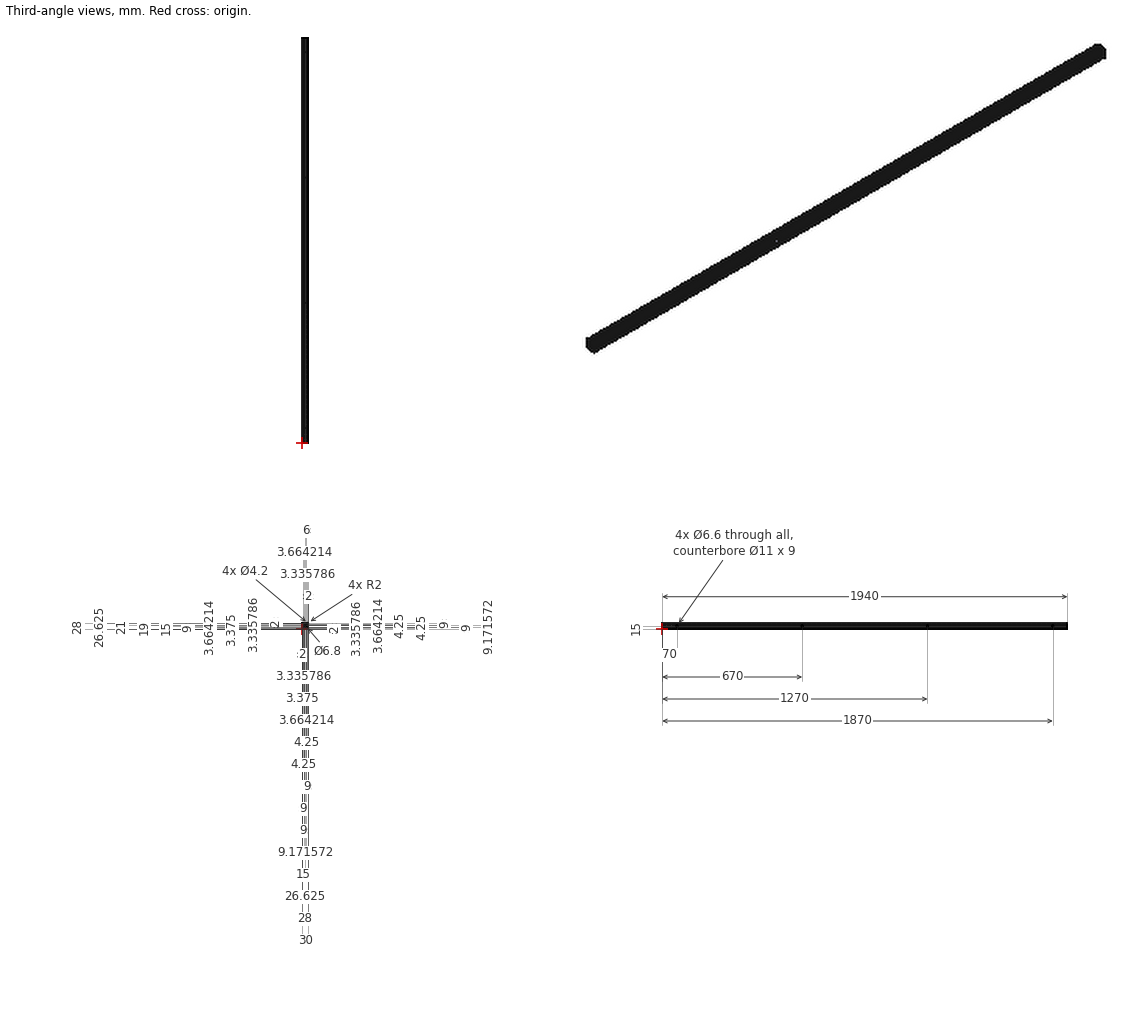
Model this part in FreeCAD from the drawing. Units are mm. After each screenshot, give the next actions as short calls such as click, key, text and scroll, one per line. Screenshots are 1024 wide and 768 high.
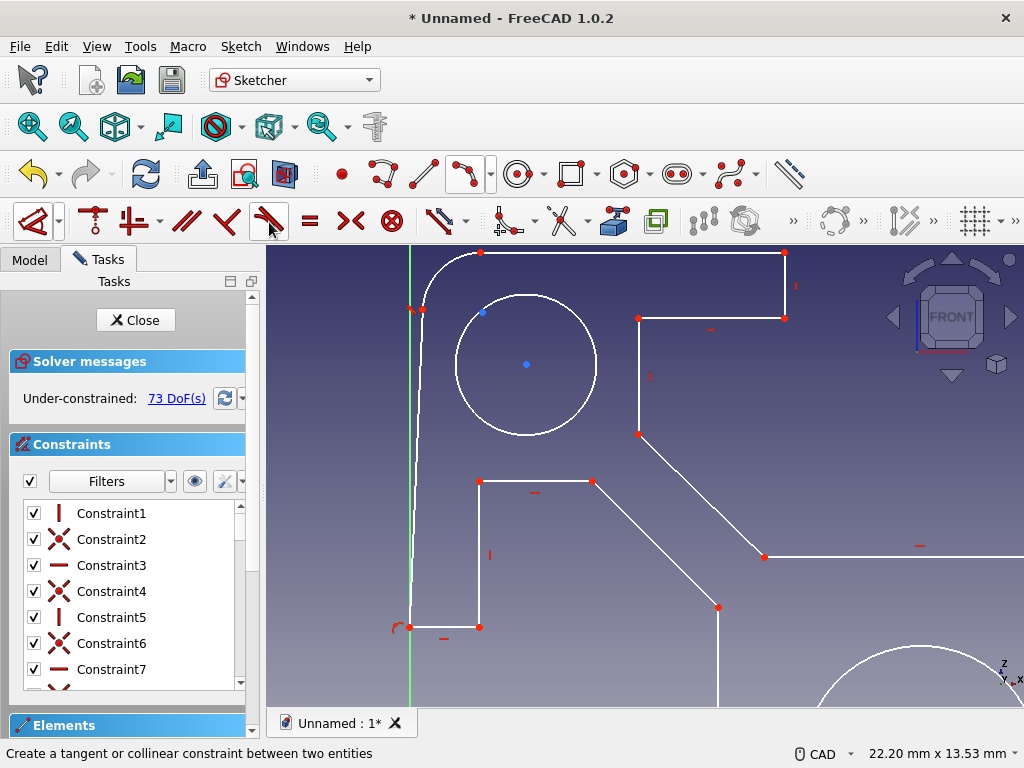
scroll(428, 354, down, 6)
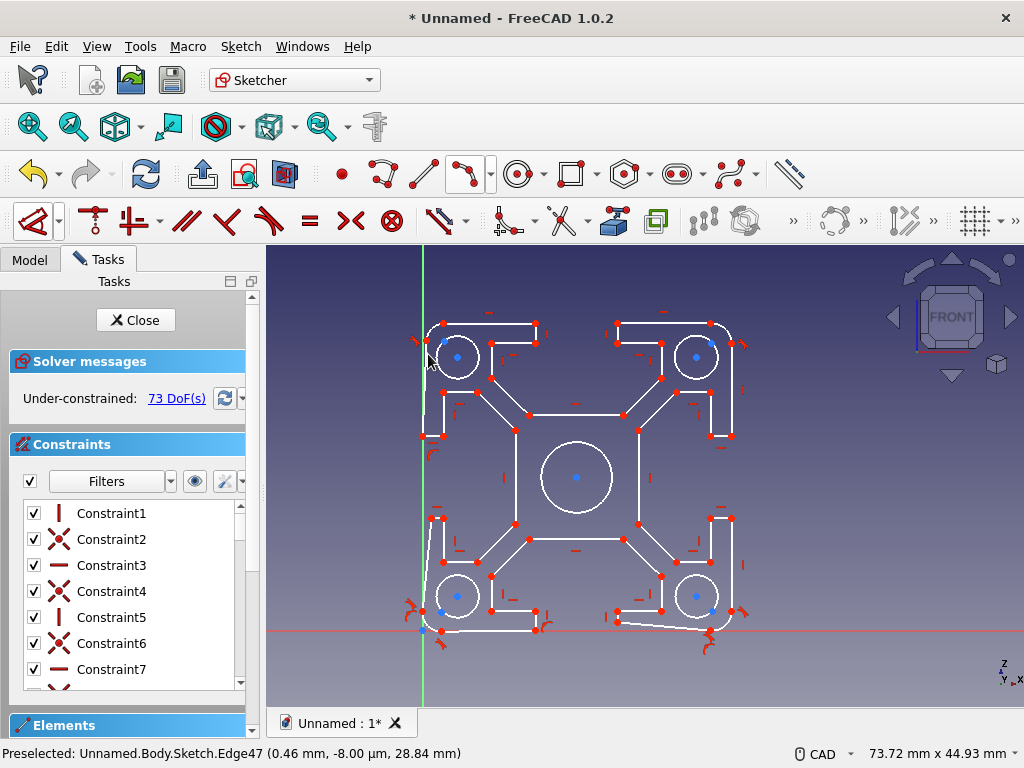
click(471, 324)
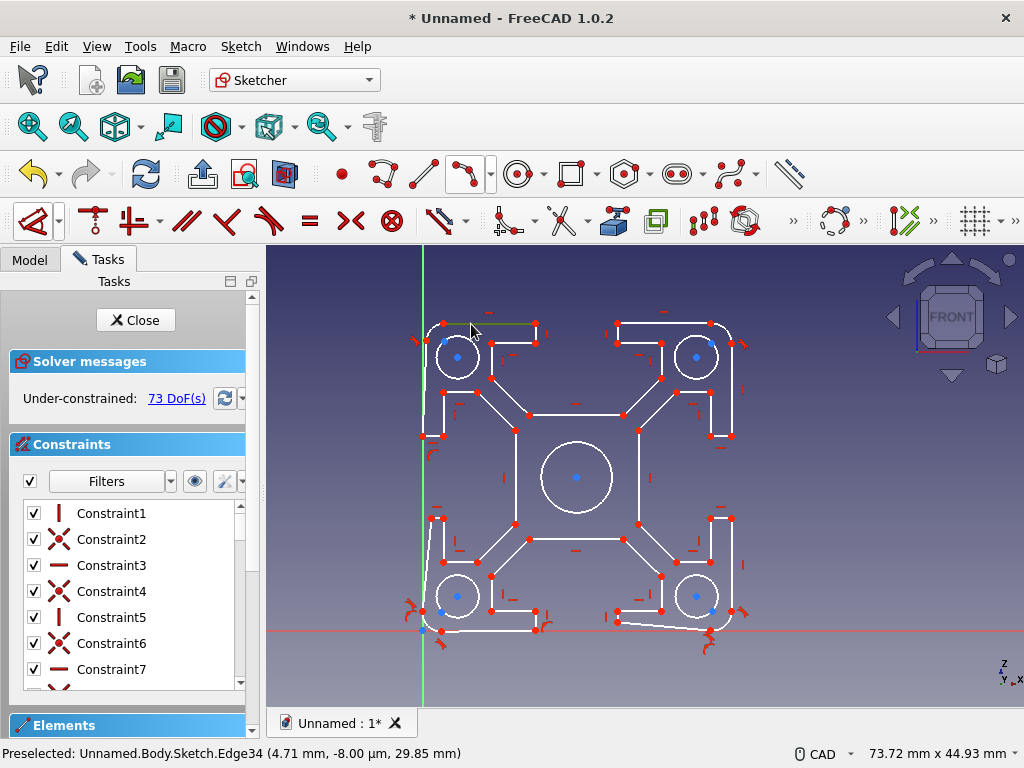
scroll(432, 329, up, 2)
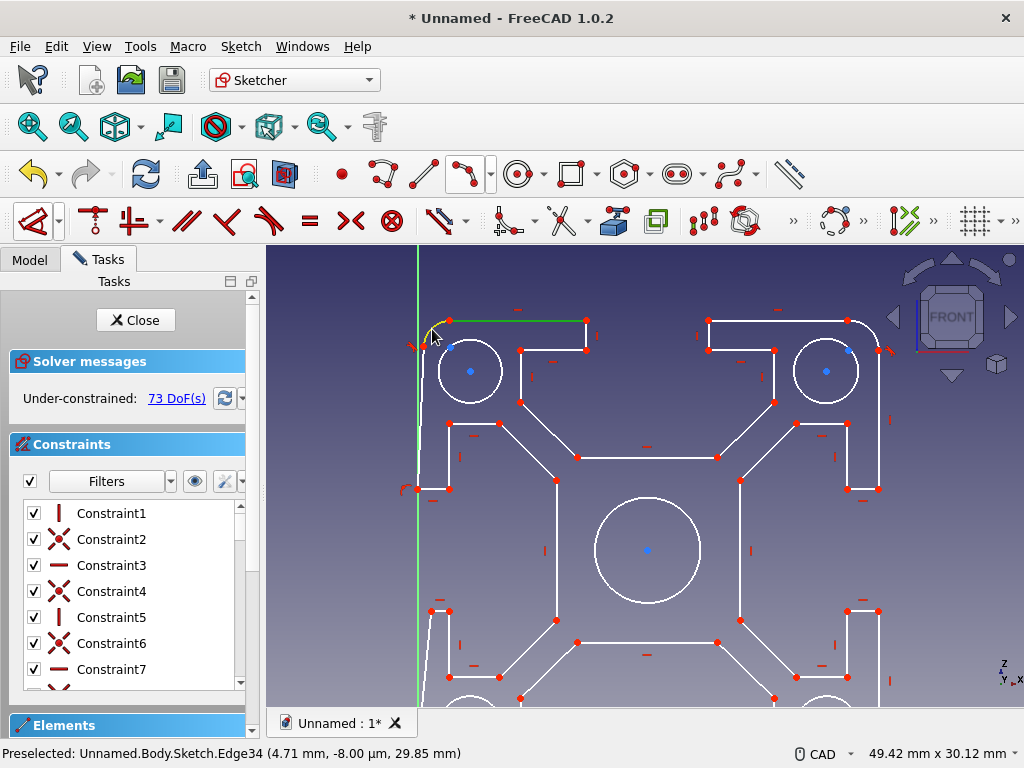
click(432, 329)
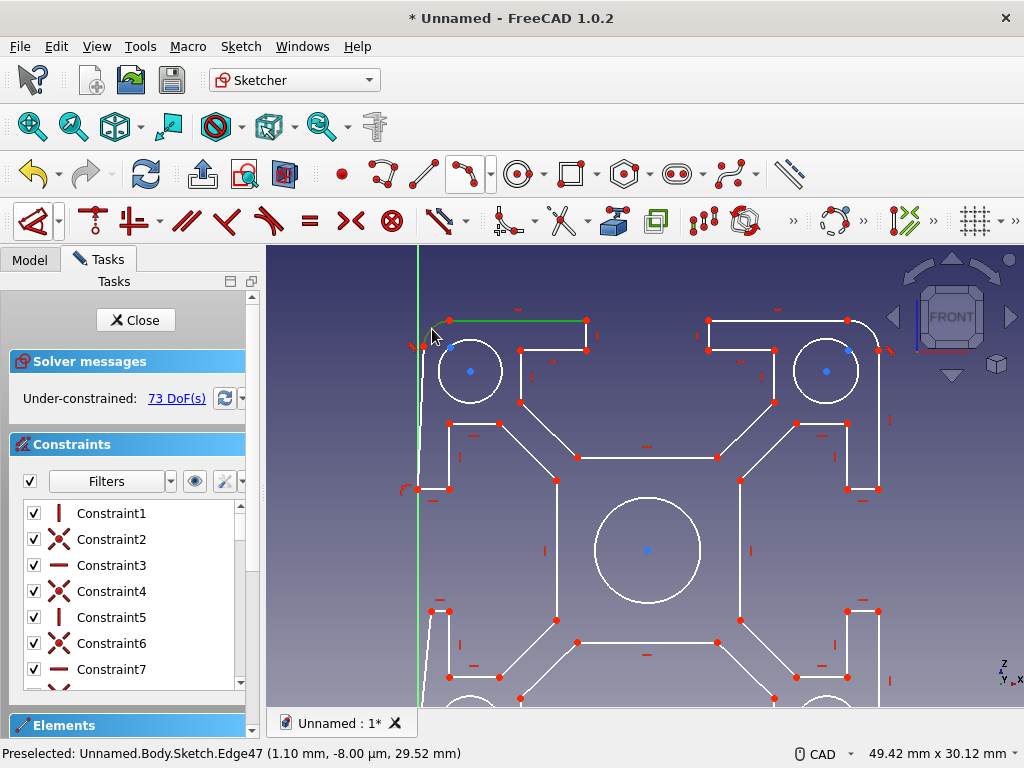
click(269, 222)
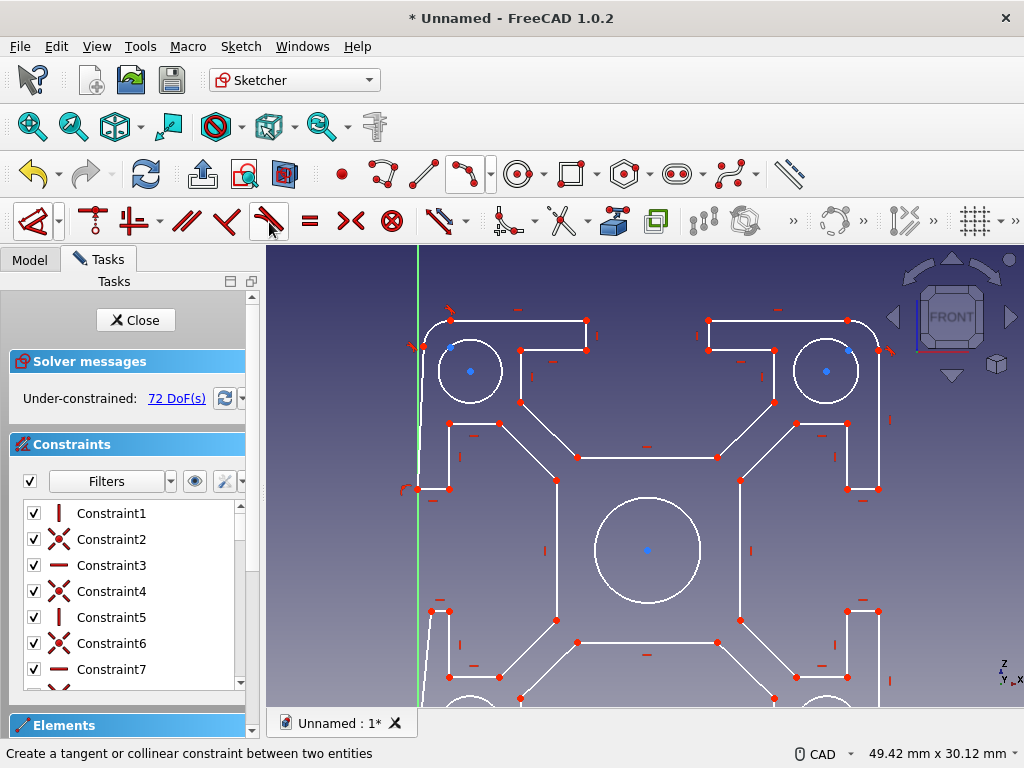
click(750, 321)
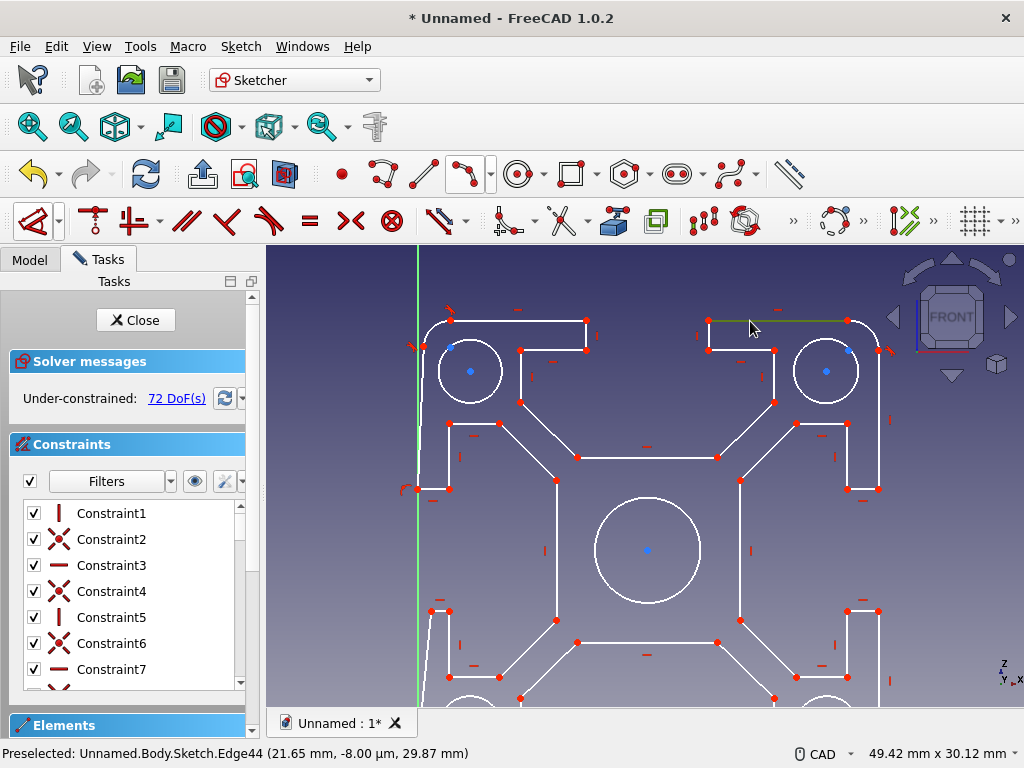
scroll(857, 322, up, 2)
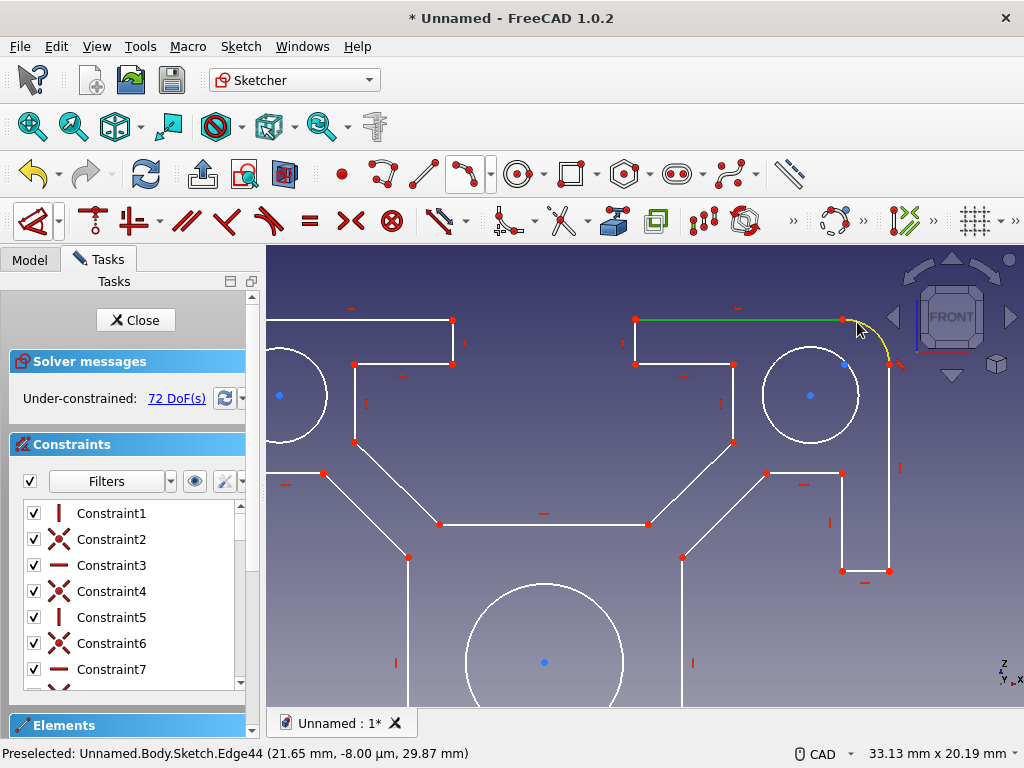
click(857, 321)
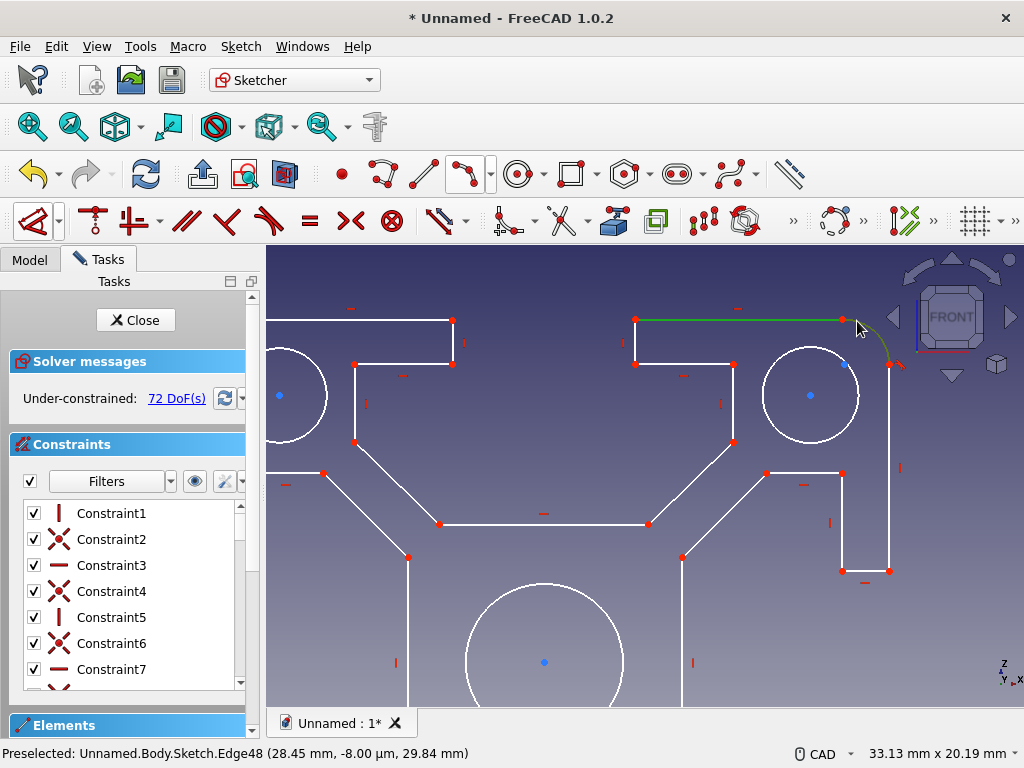
key(t)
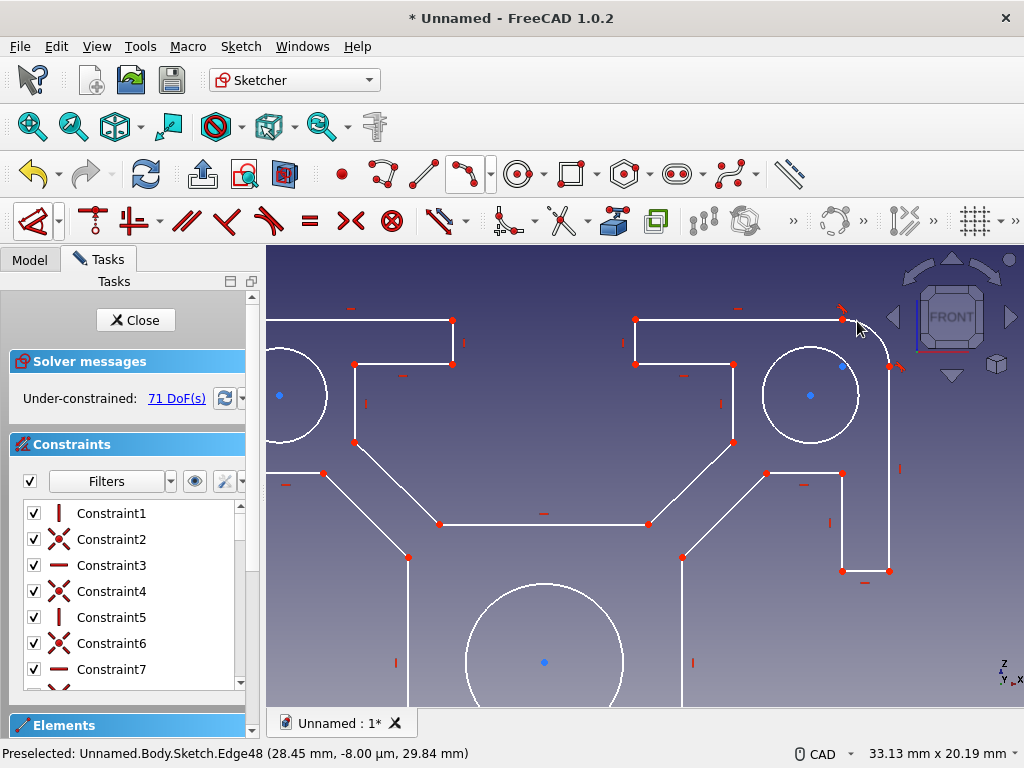
scroll(602, 326, down, 4)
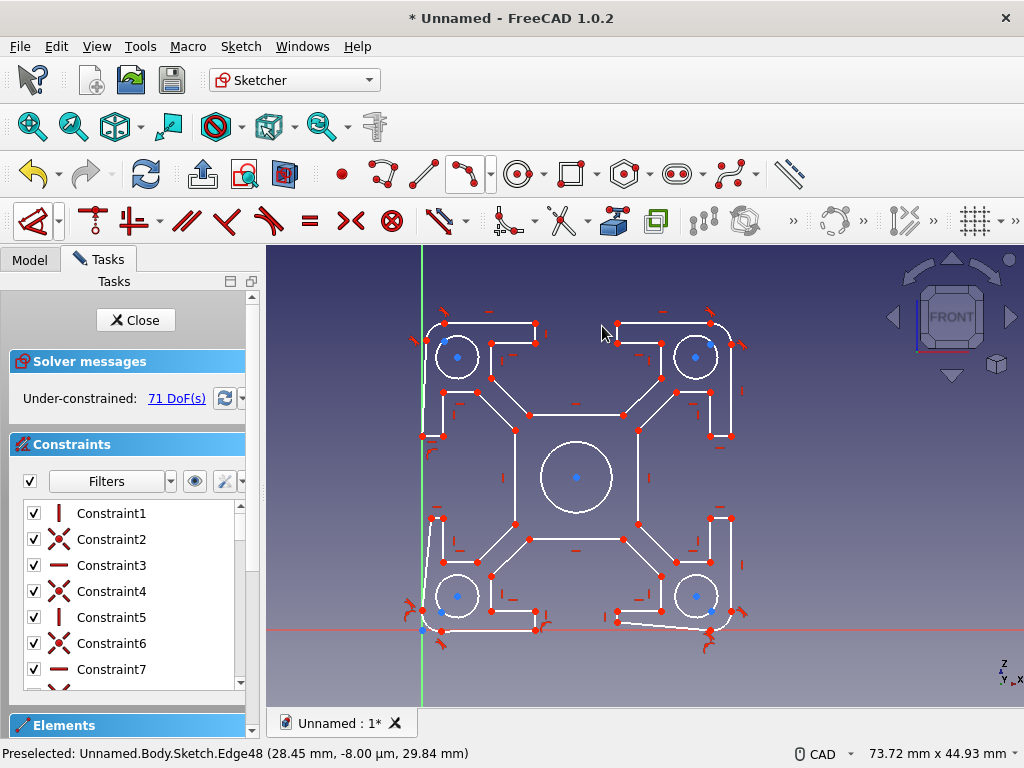
scroll(645, 625, up, 5)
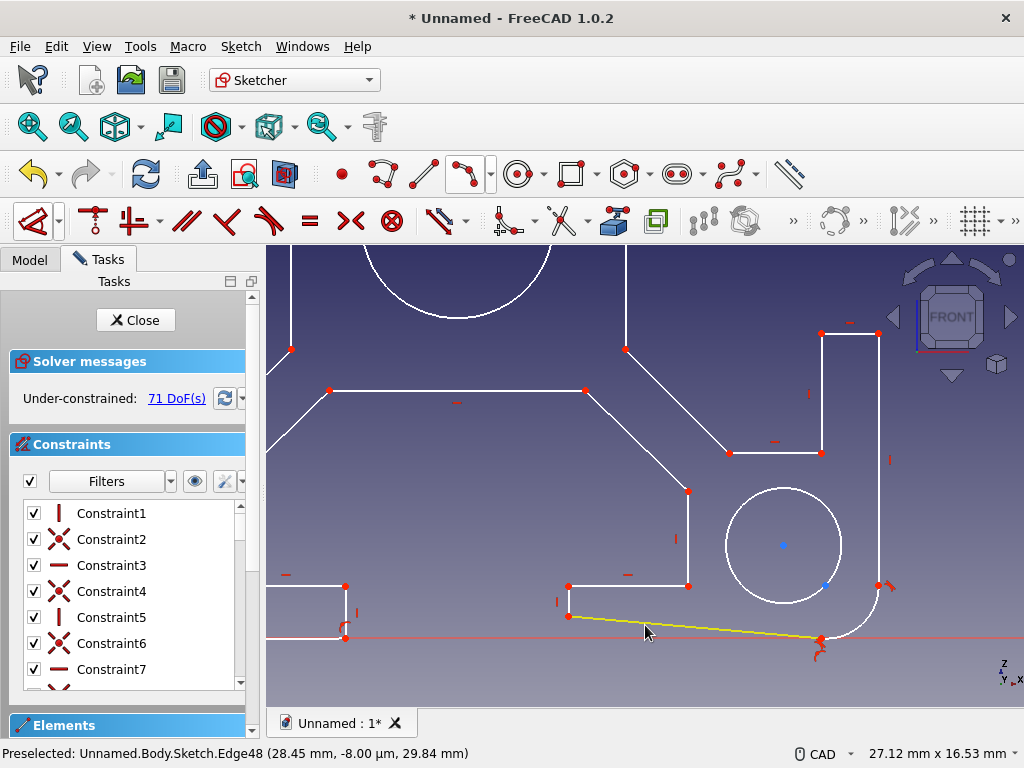
click(644, 623)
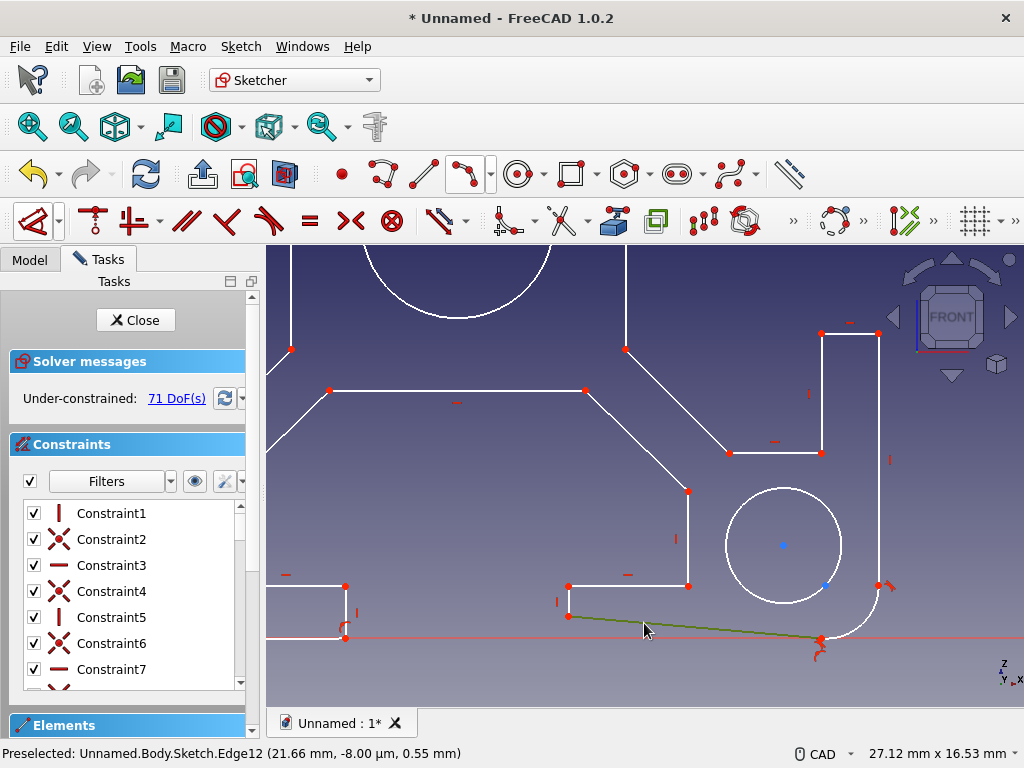
key(h)